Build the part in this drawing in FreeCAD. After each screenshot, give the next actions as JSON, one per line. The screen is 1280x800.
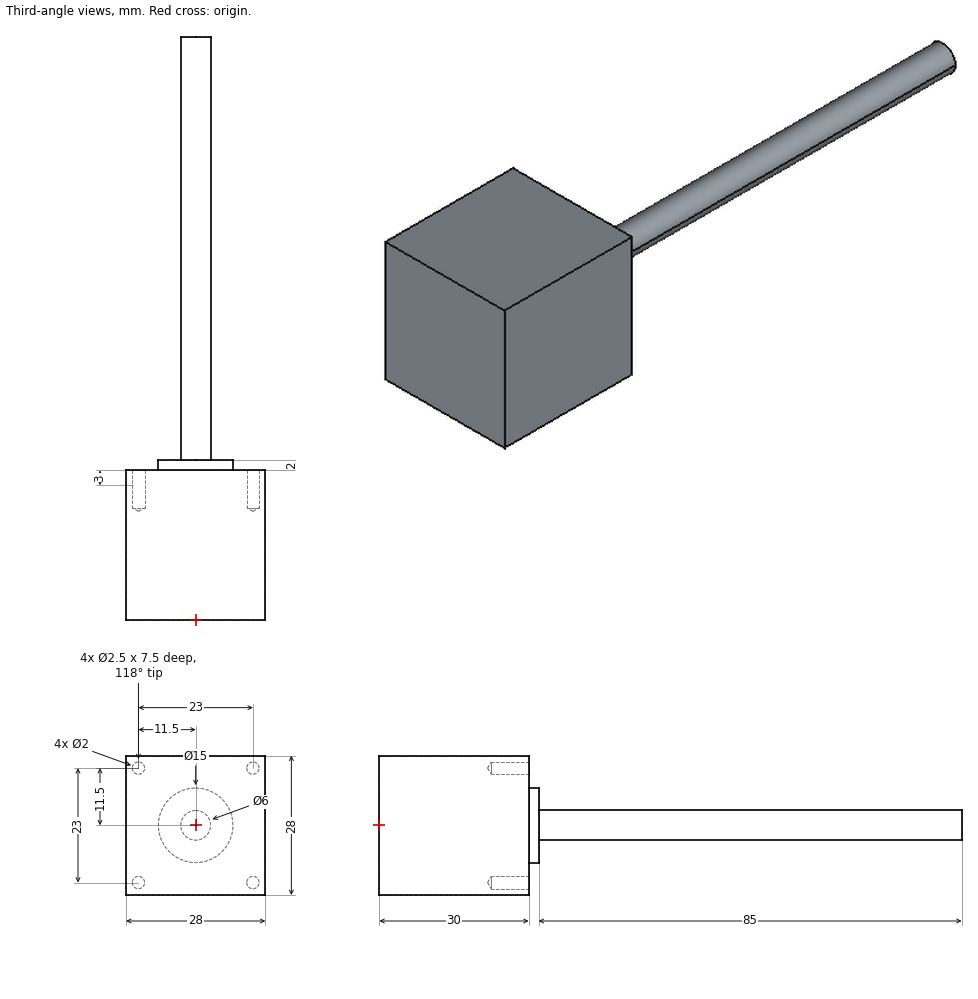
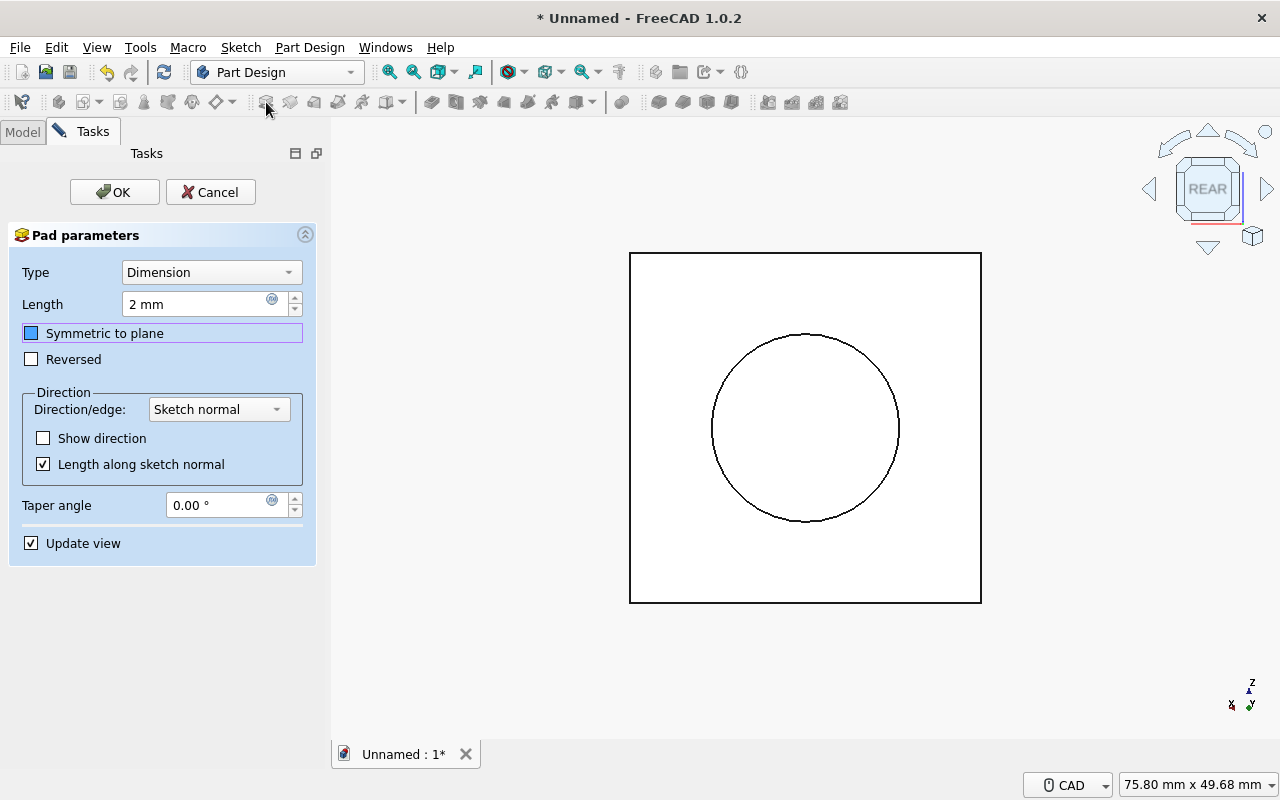
{"action": "left_click", "coordinate": [115, 192]}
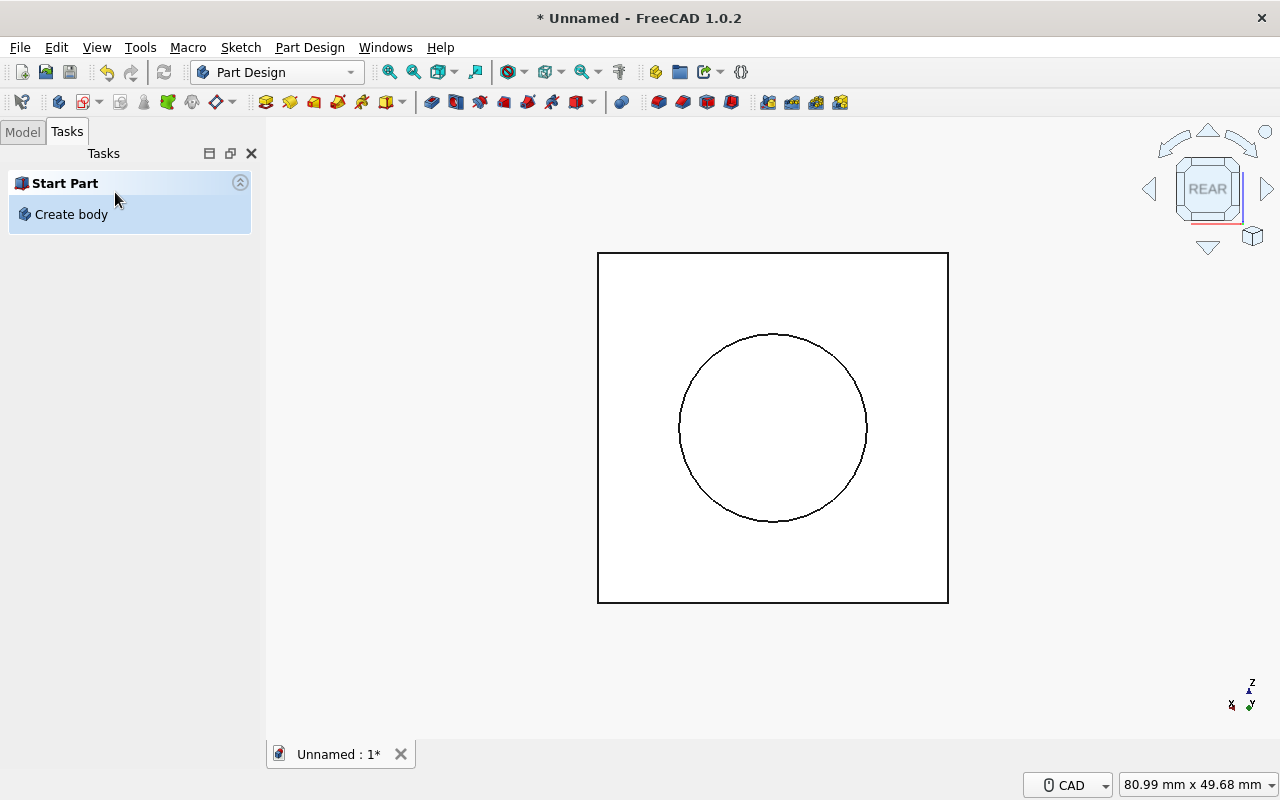
{"action": "left_click", "coordinate": [773, 427]}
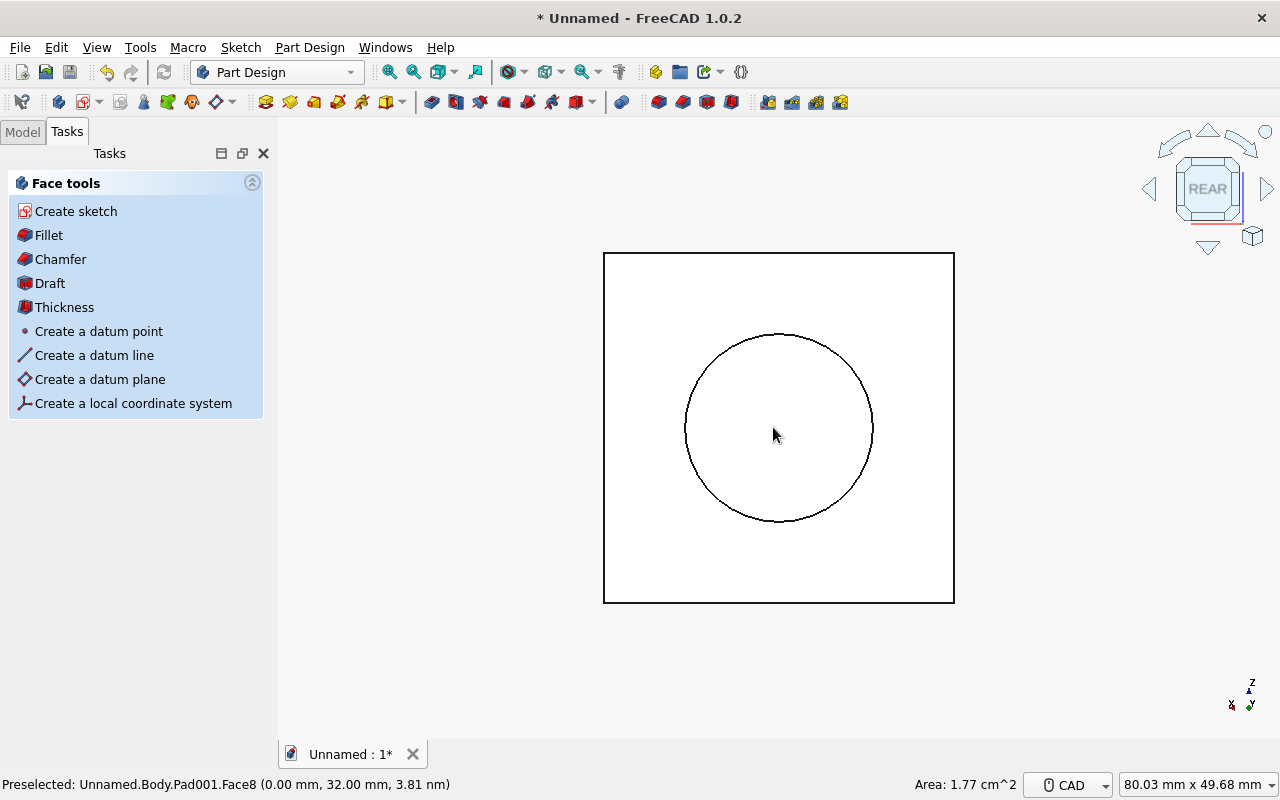
{"action": "left_click", "coordinate": [84, 102]}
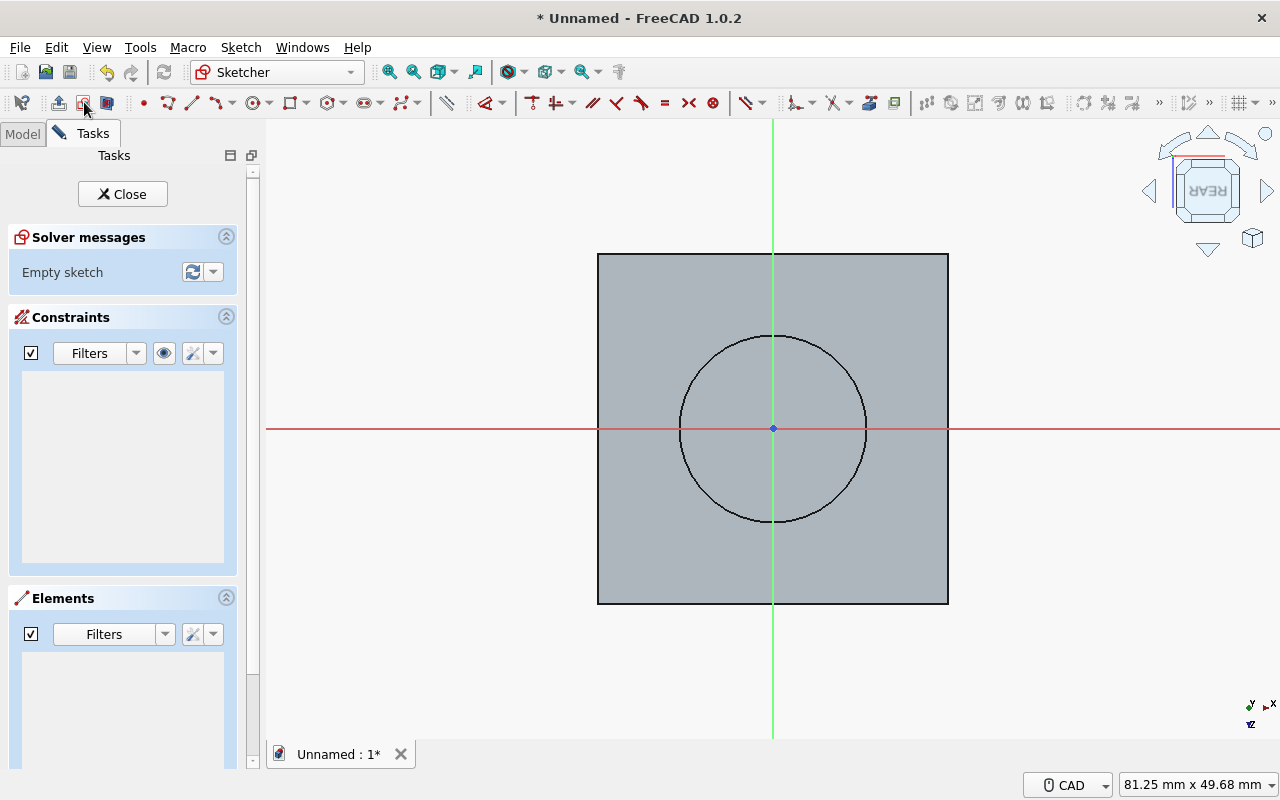
{"action": "scroll", "coordinate": [790, 429], "scroll_direction": "up", "scroll_amount": 8}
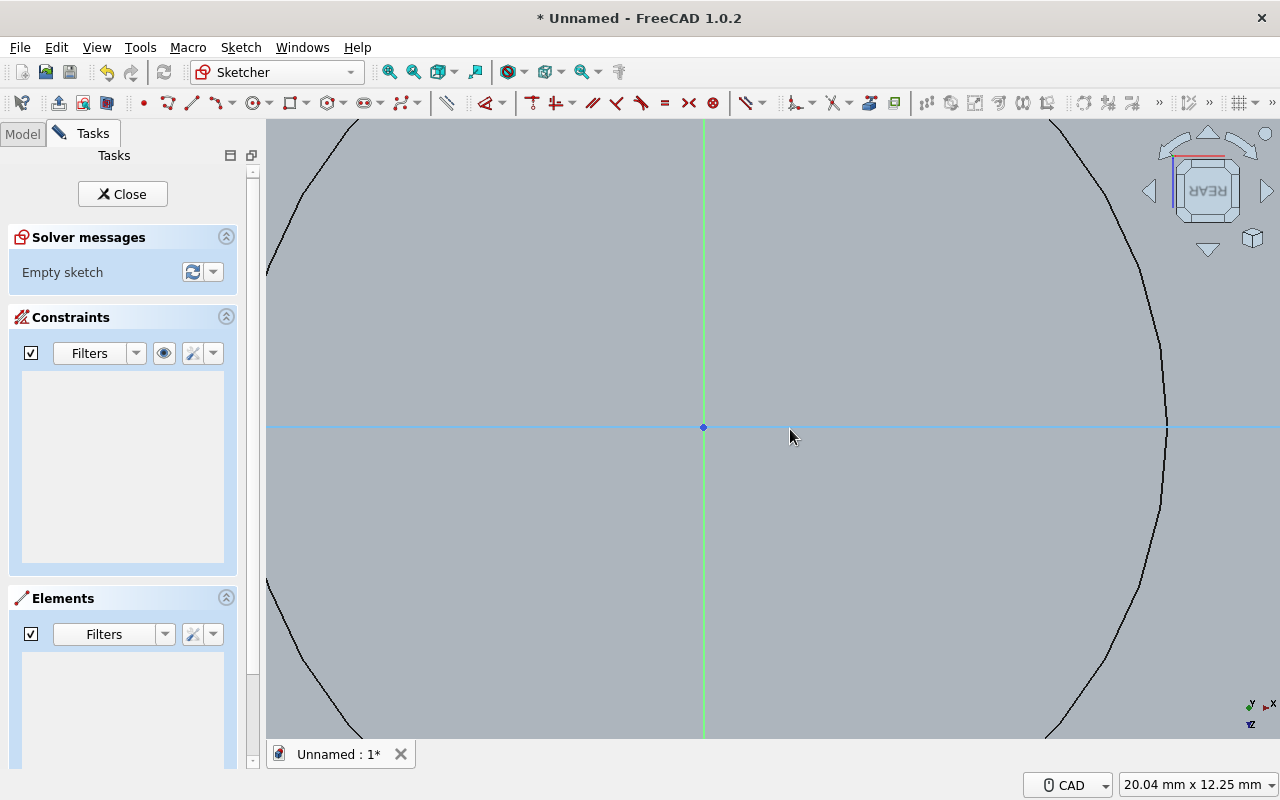
{"action": "left_click", "coordinate": [254, 104]}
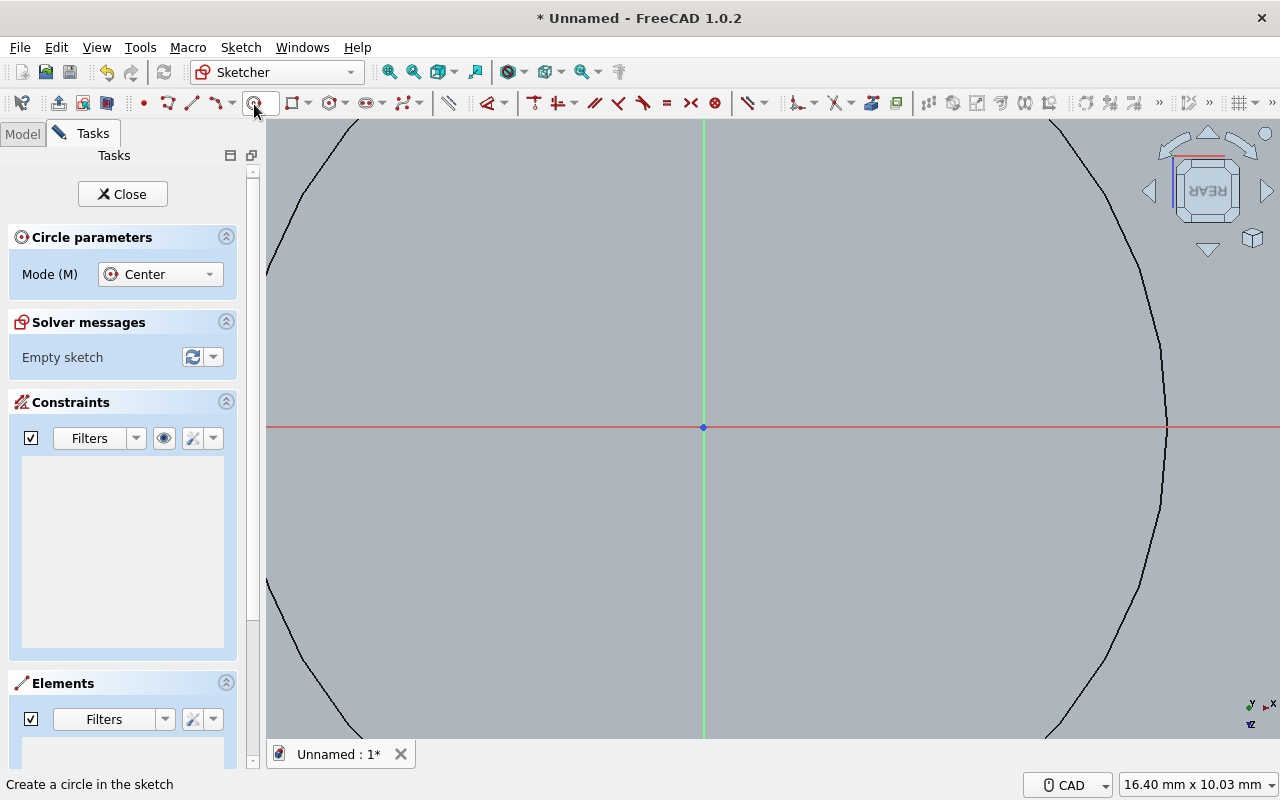
{"action": "left_click", "coordinate": [704, 427]}
{"action": "left_click", "coordinate": [835, 296]}
{"action": "key", "text": "Escape"}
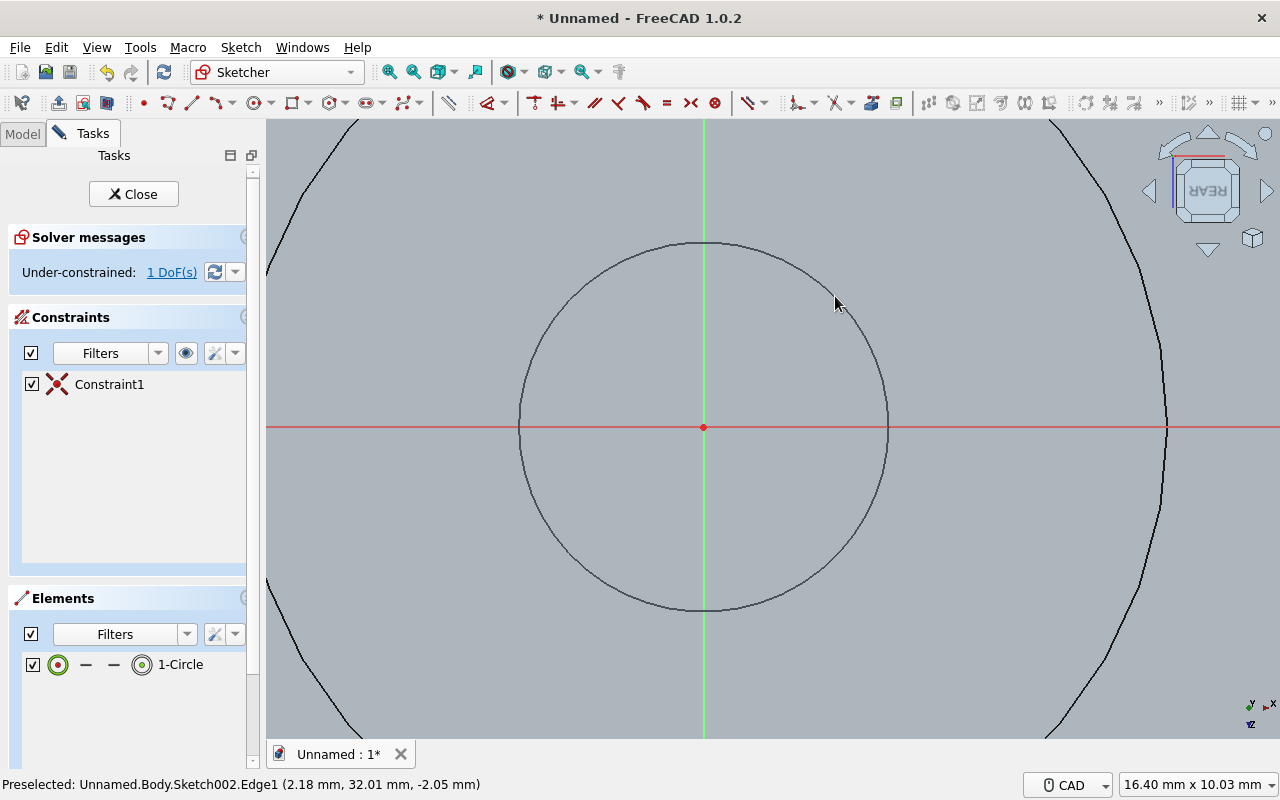
{"action": "left_click", "coordinate": [488, 104]}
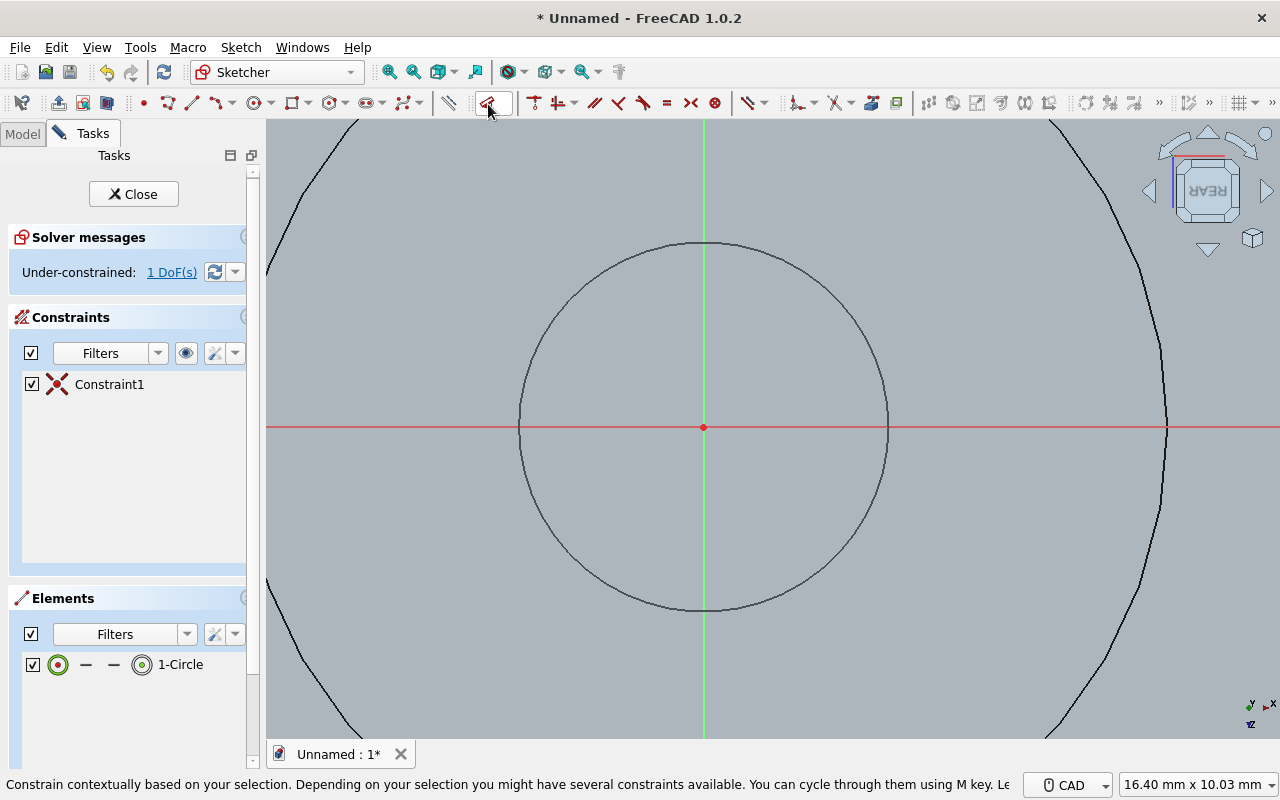
{"action": "left_click", "coordinate": [834, 296]}
{"action": "left_click", "coordinate": [857, 273]}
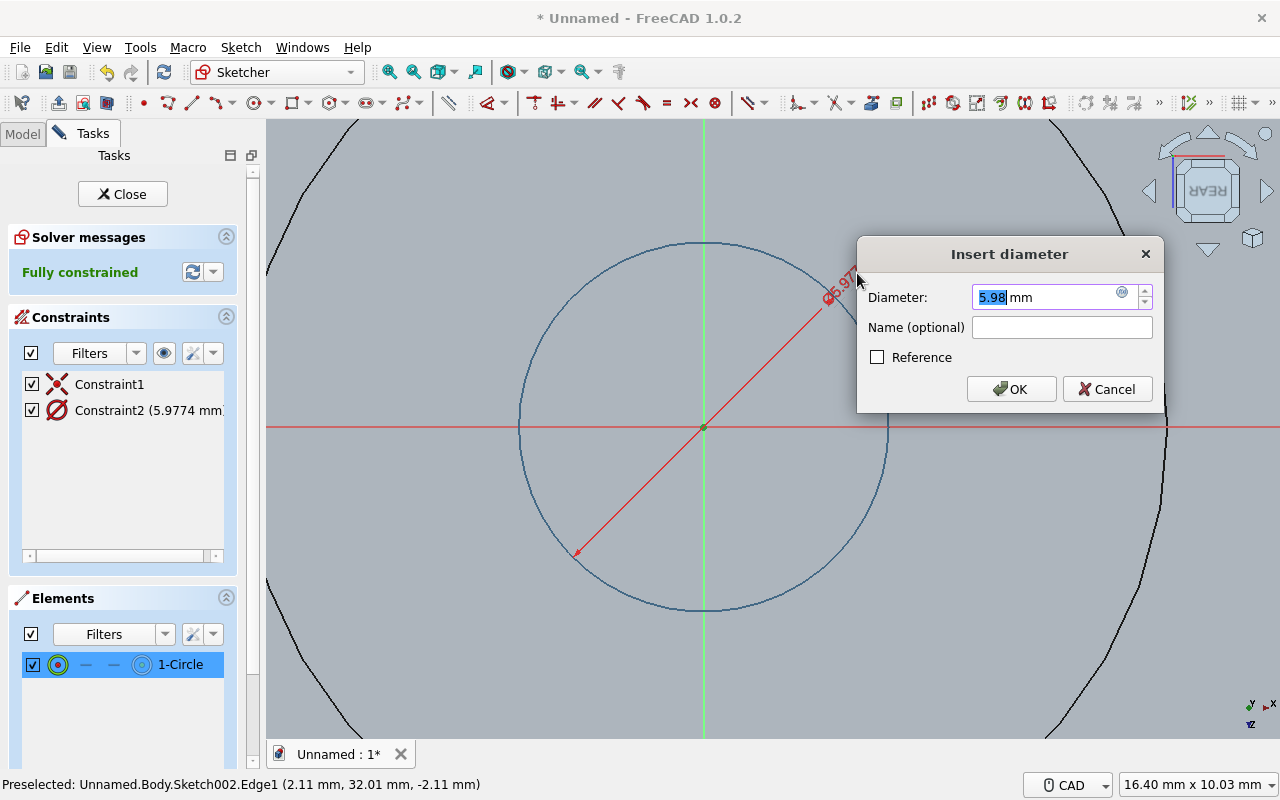
{"action": "type", "text": "6"}
{"action": "key", "text": "Return"}
{"action": "key", "text": "Escape"}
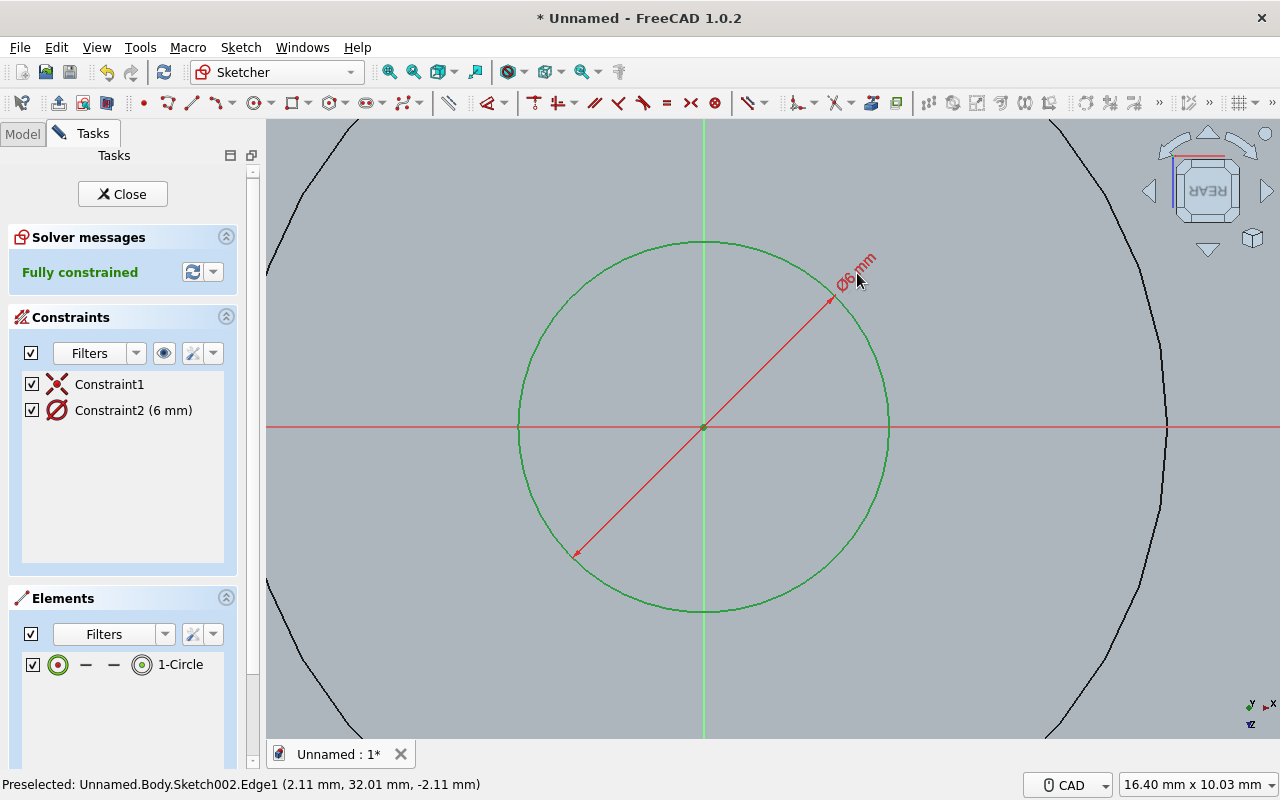
{"action": "left_click", "coordinate": [123, 194]}